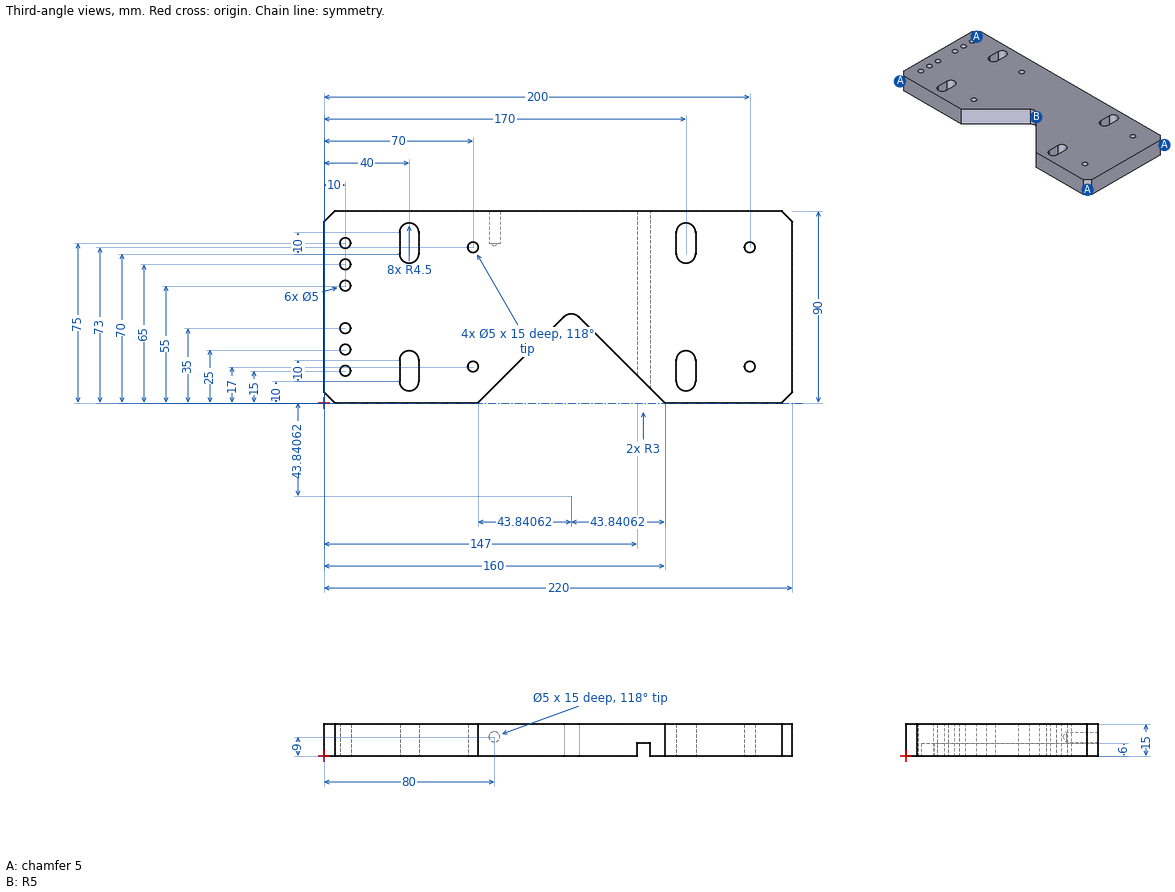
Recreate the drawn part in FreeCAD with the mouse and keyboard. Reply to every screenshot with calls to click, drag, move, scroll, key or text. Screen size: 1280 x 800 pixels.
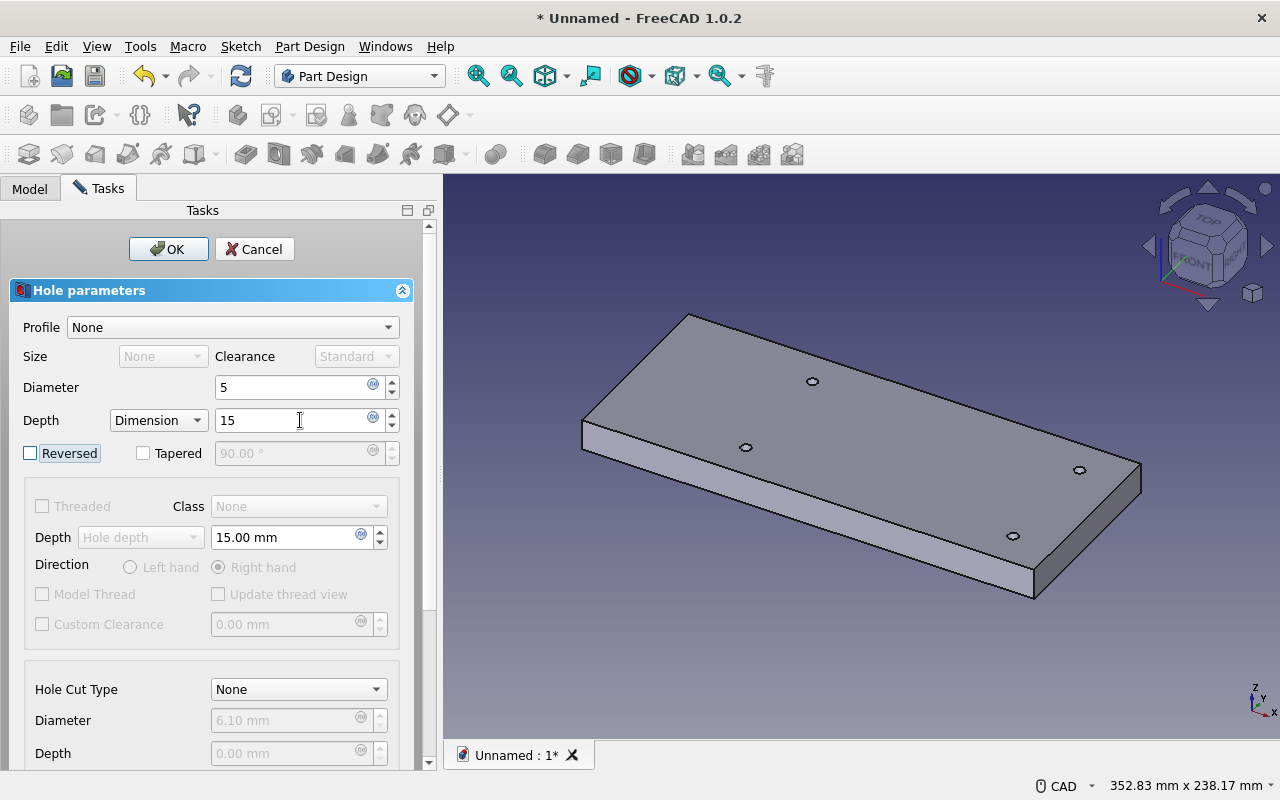
click(169, 249)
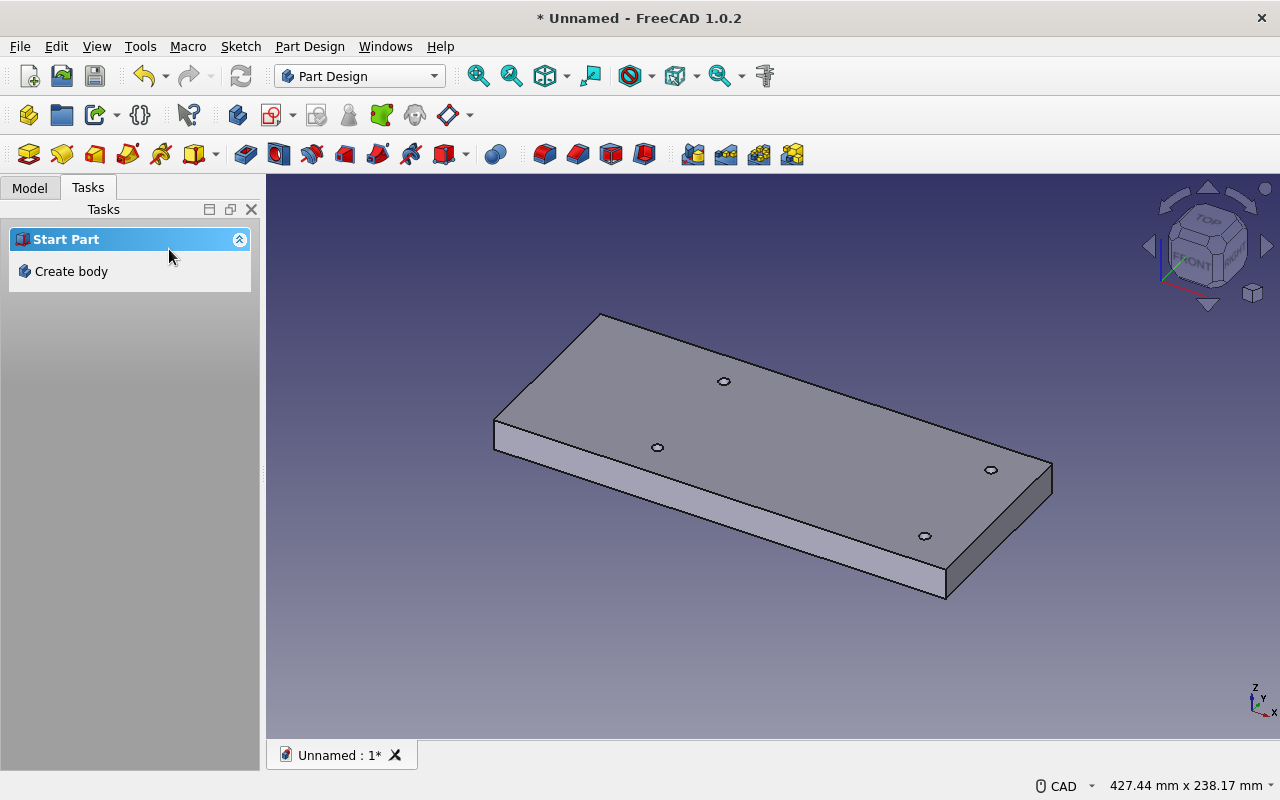
click(838, 462)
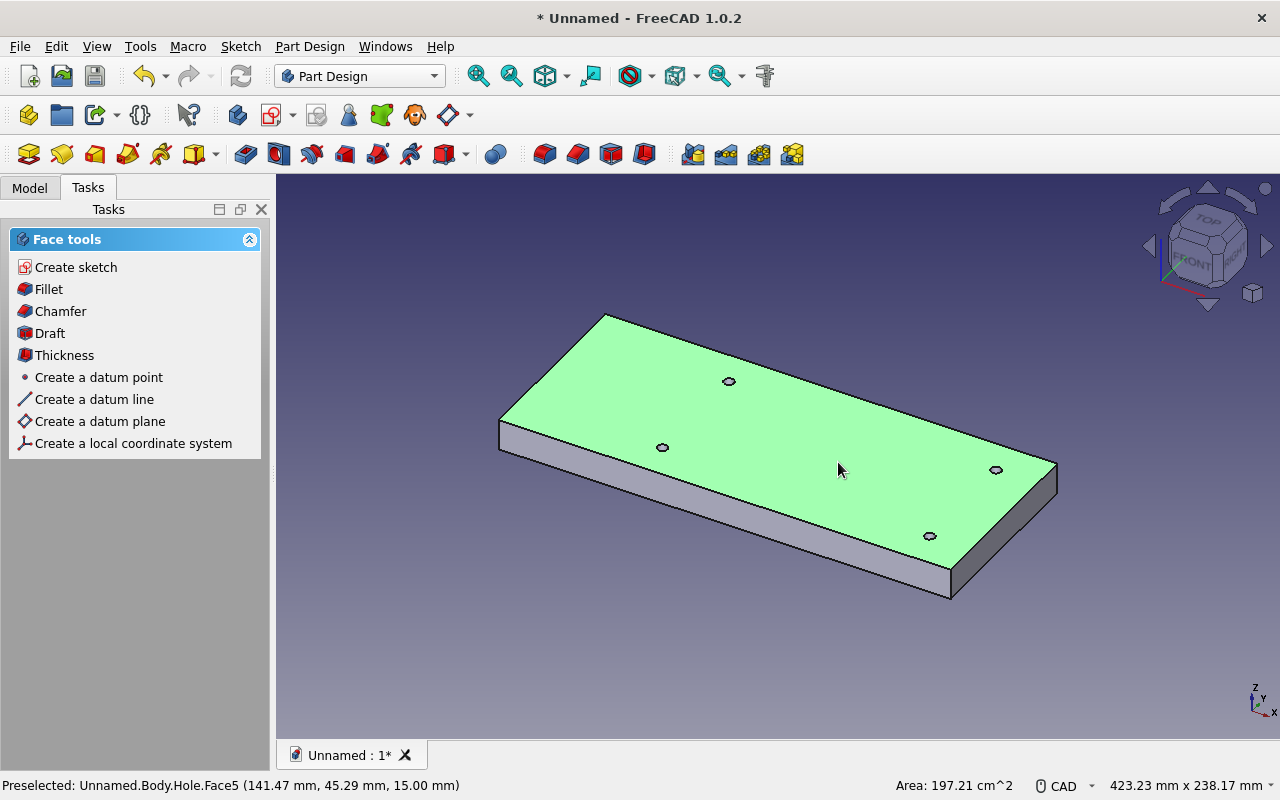
click(270, 116)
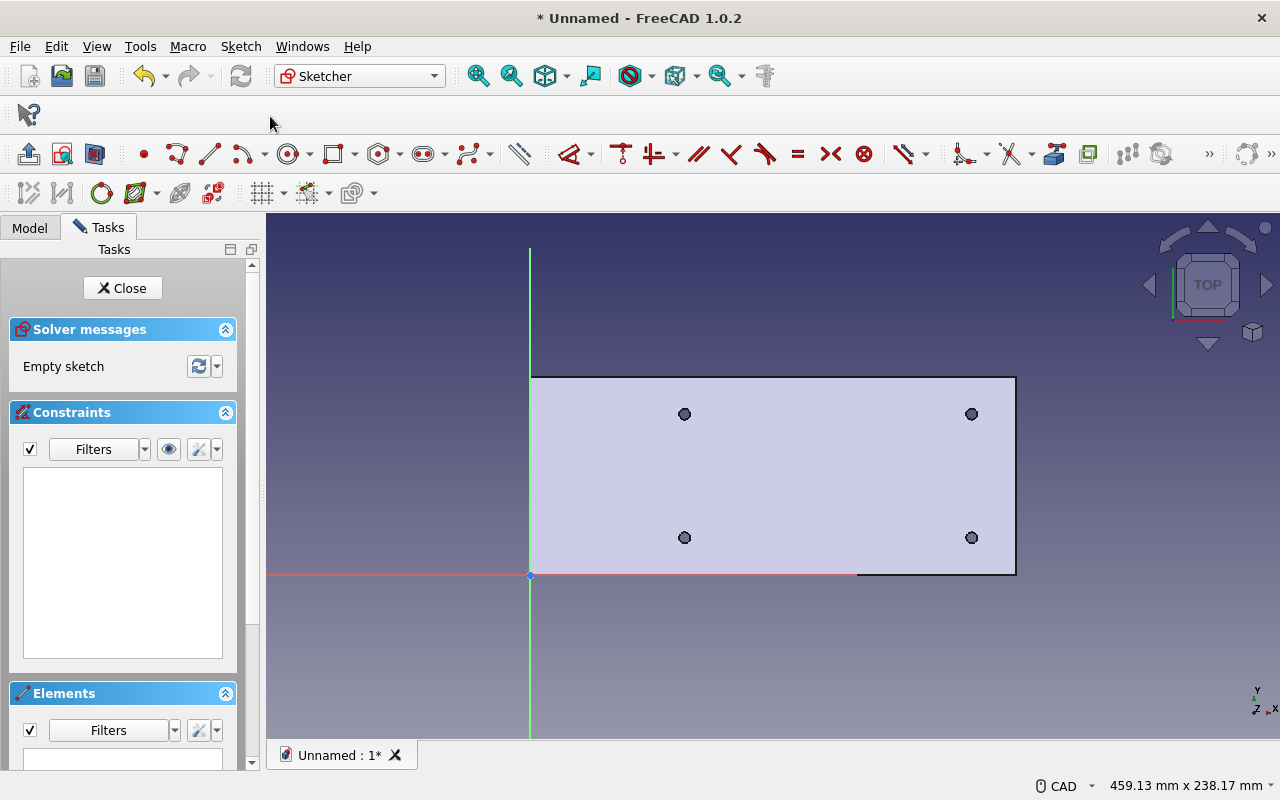
scroll(760, 494, up, 2)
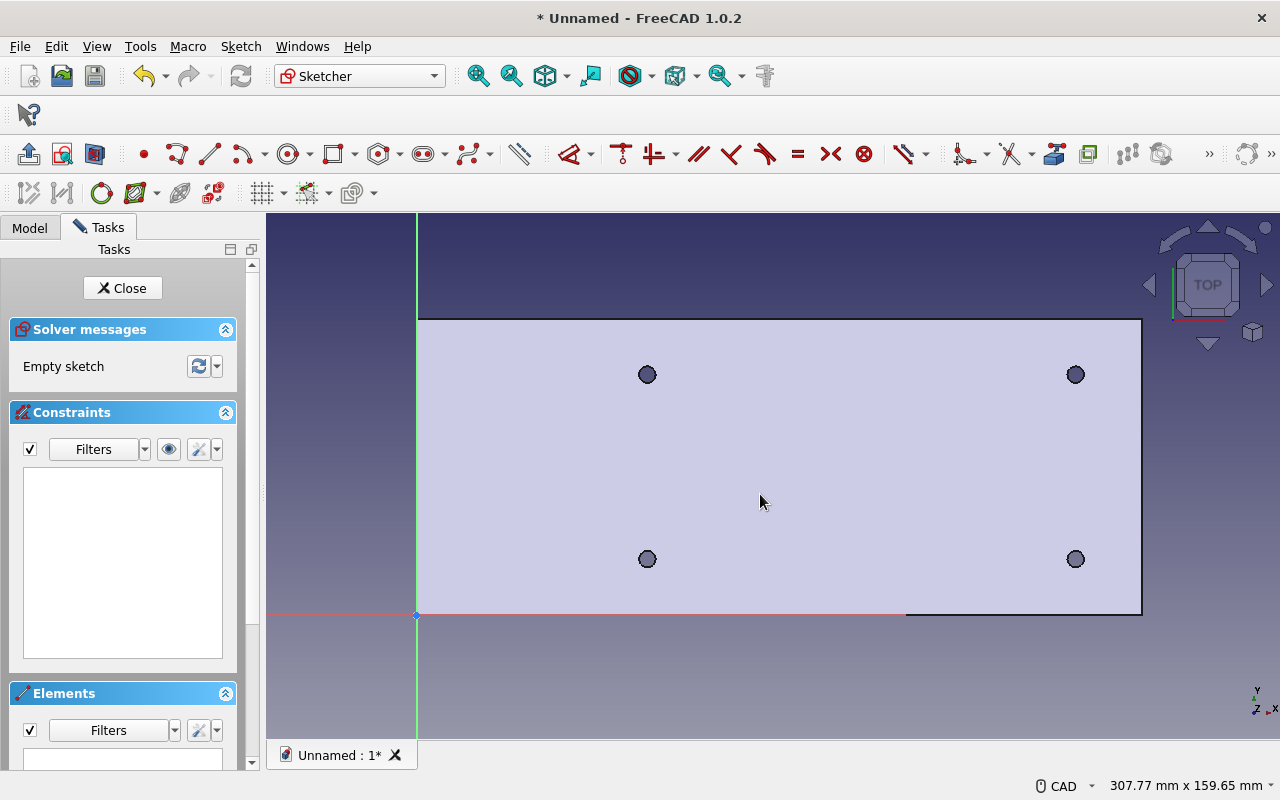
click(422, 154)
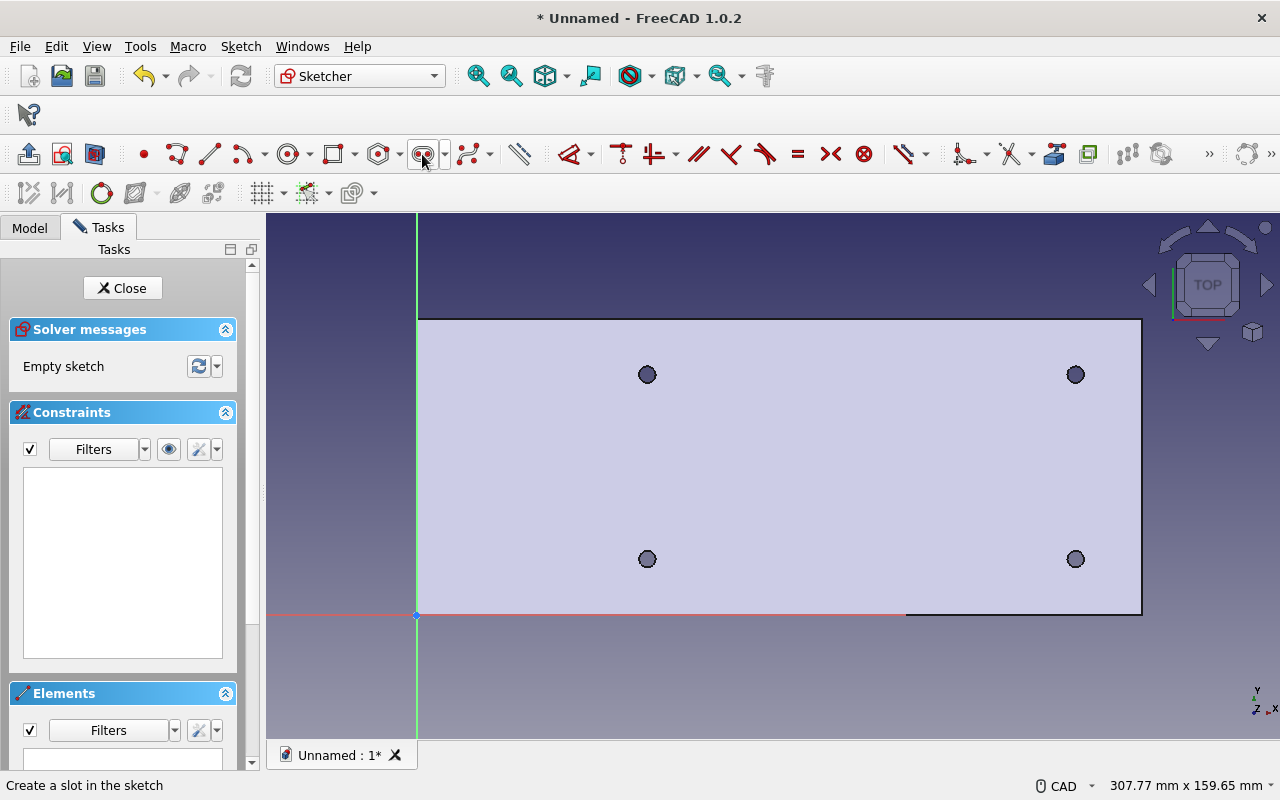
scroll(549, 385, up, 3)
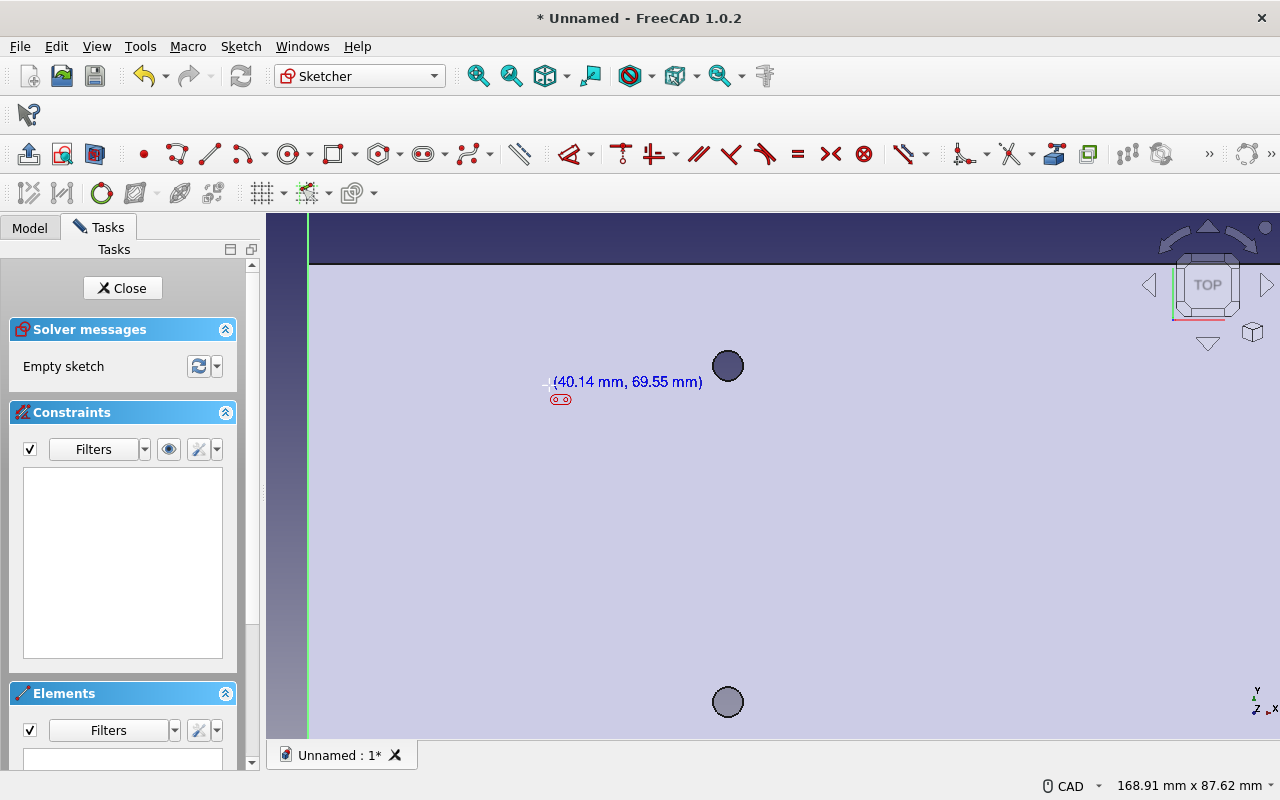
click(548, 384)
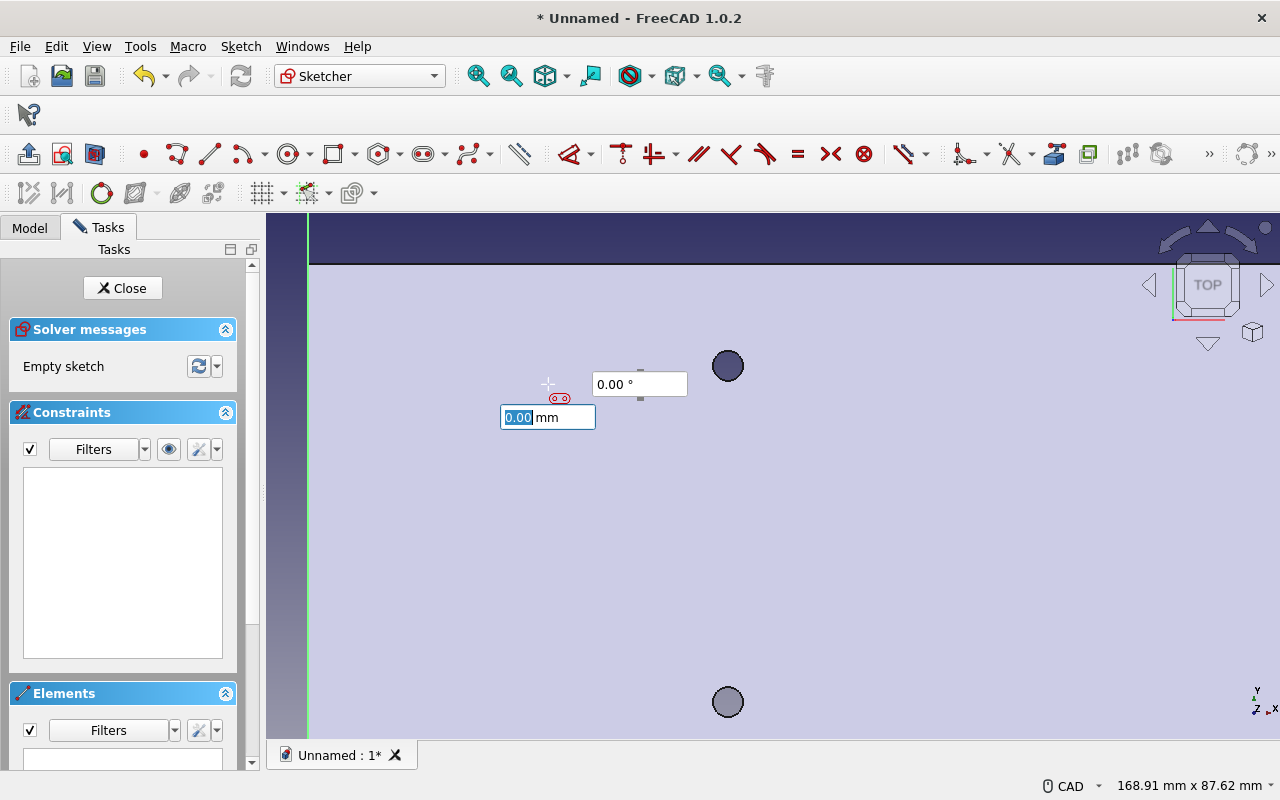
click(548, 324)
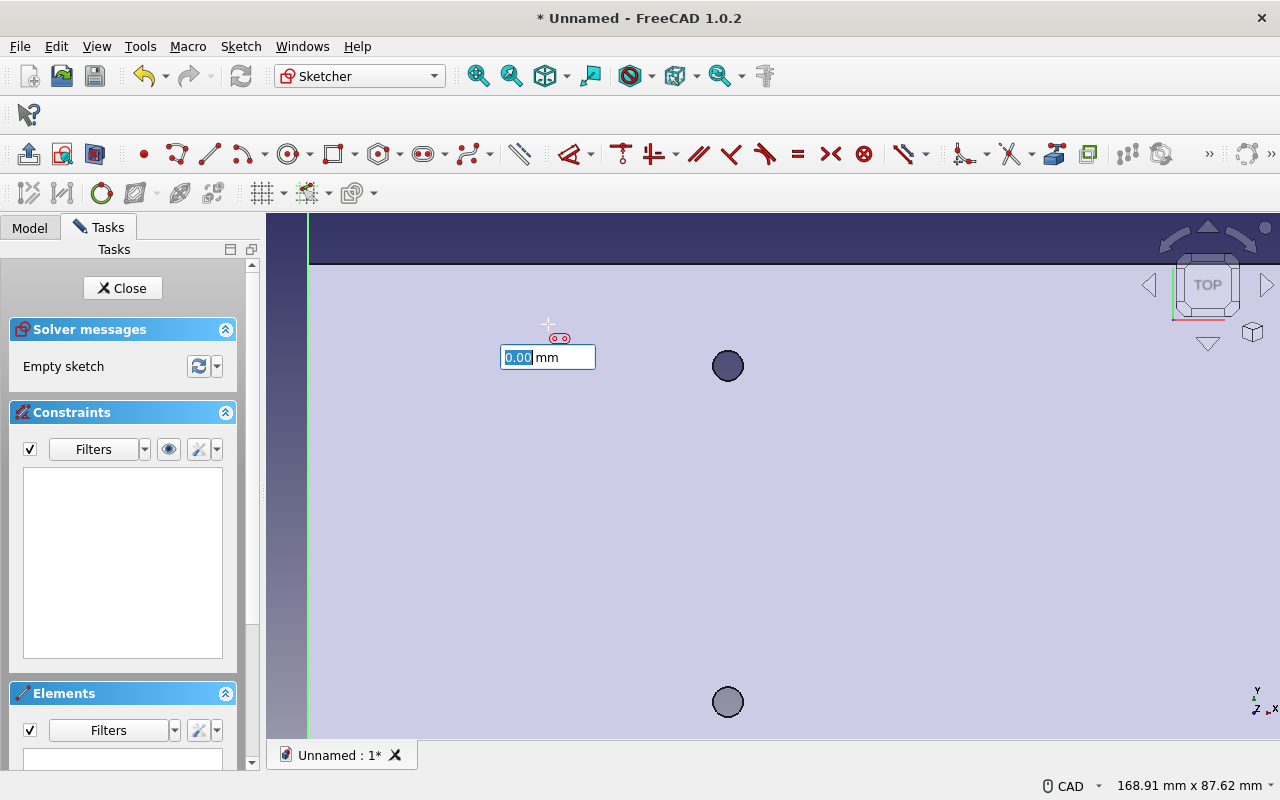
click(575, 354)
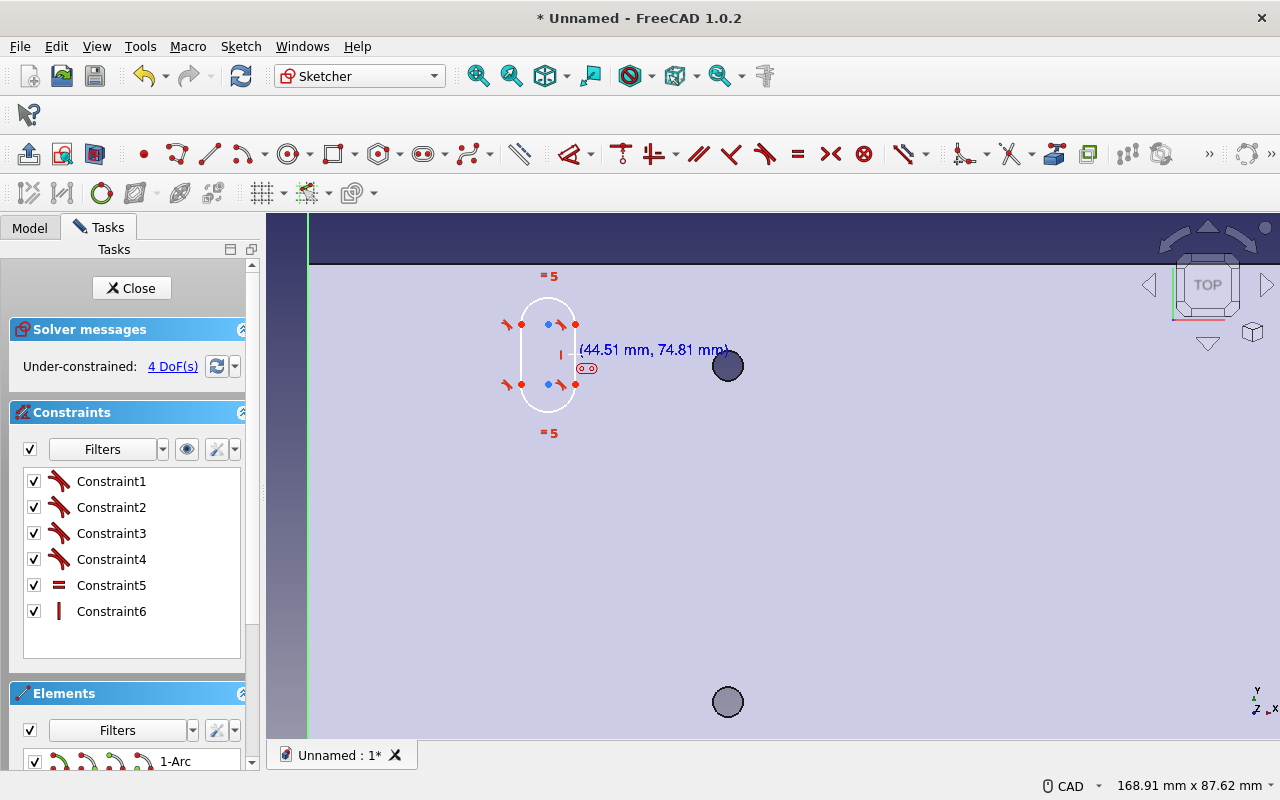
scroll(550, 385, down, 3)